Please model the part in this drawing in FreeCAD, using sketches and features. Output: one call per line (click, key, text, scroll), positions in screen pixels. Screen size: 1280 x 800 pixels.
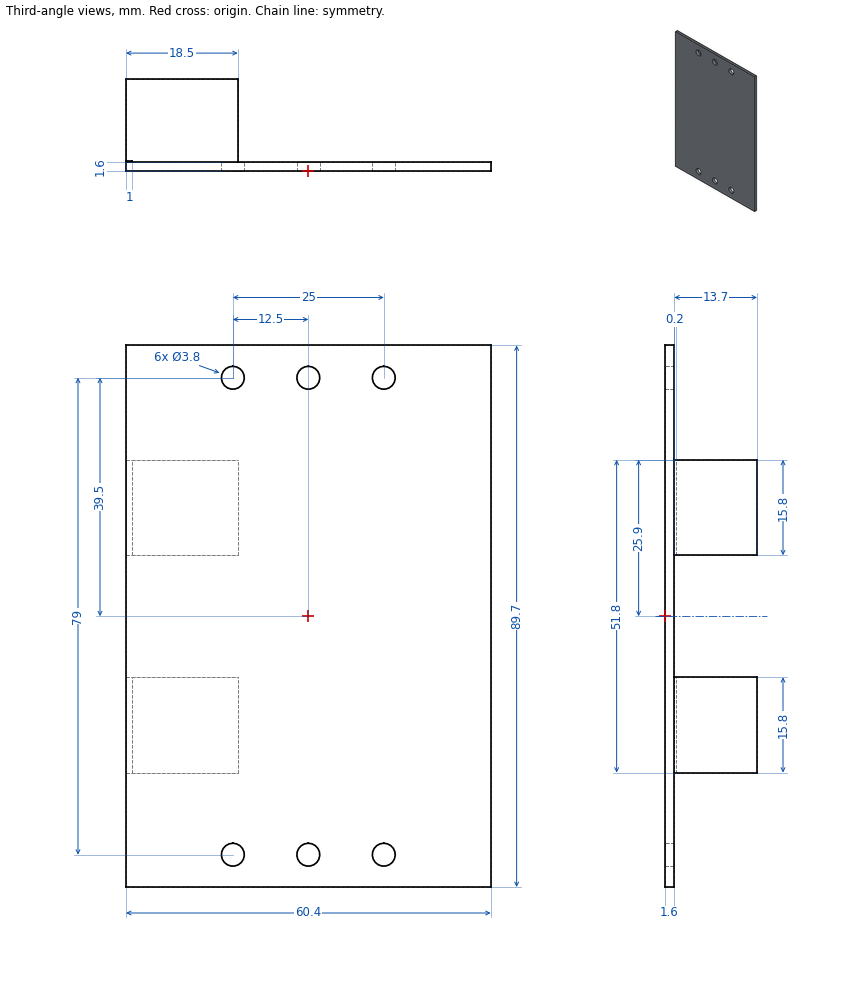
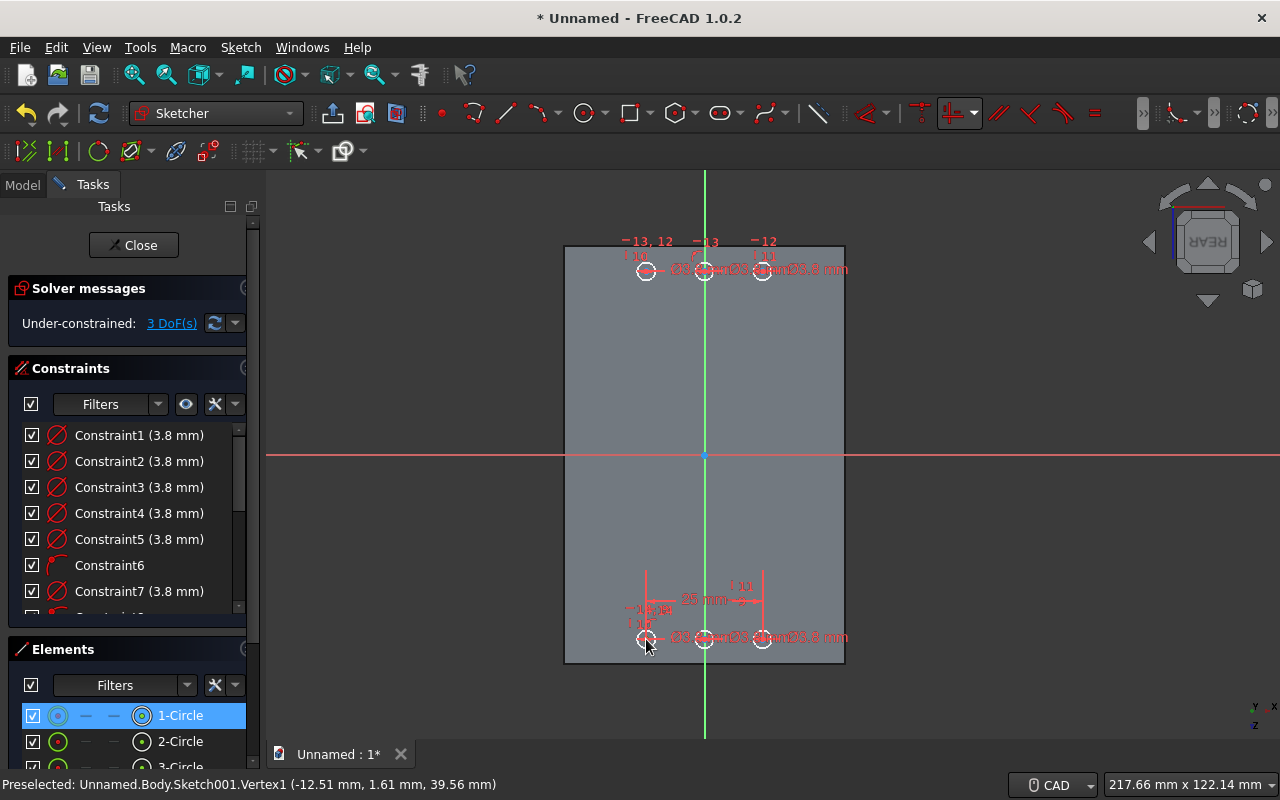
click(646, 271)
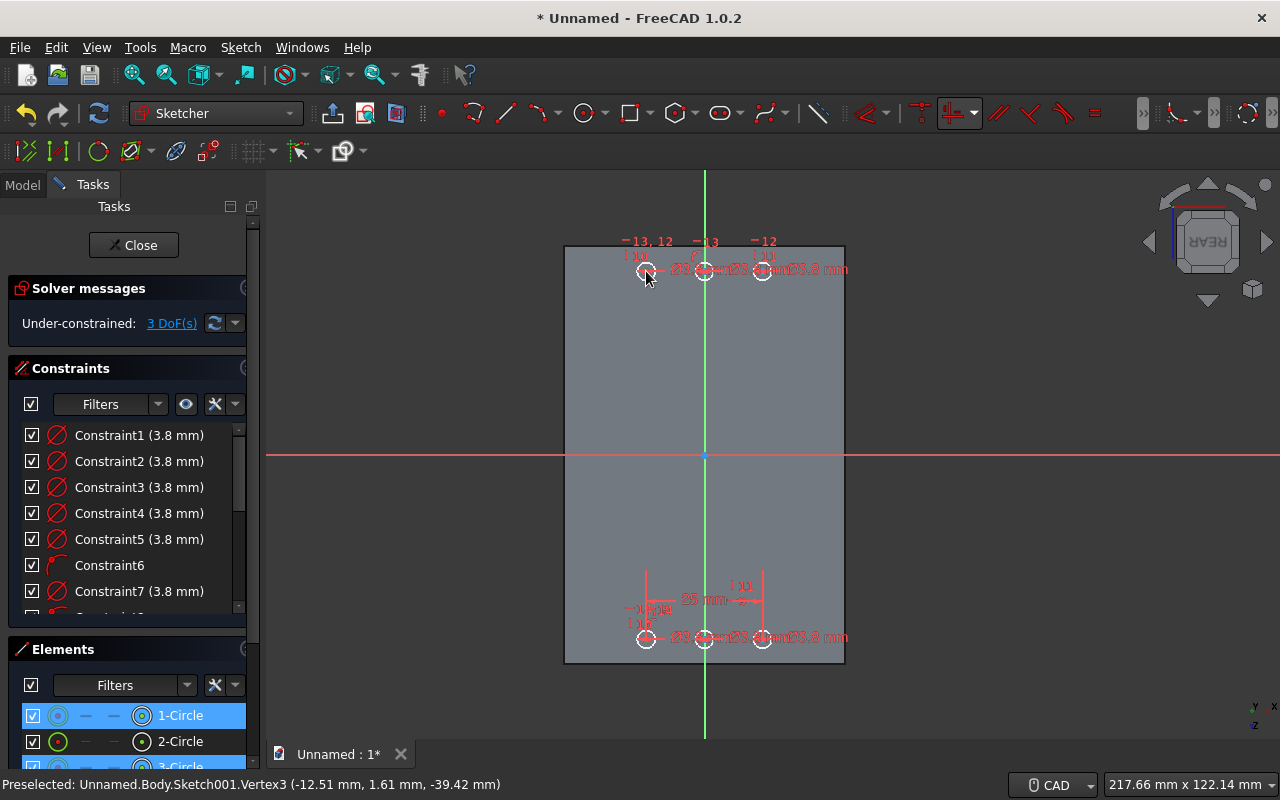
click(888, 114)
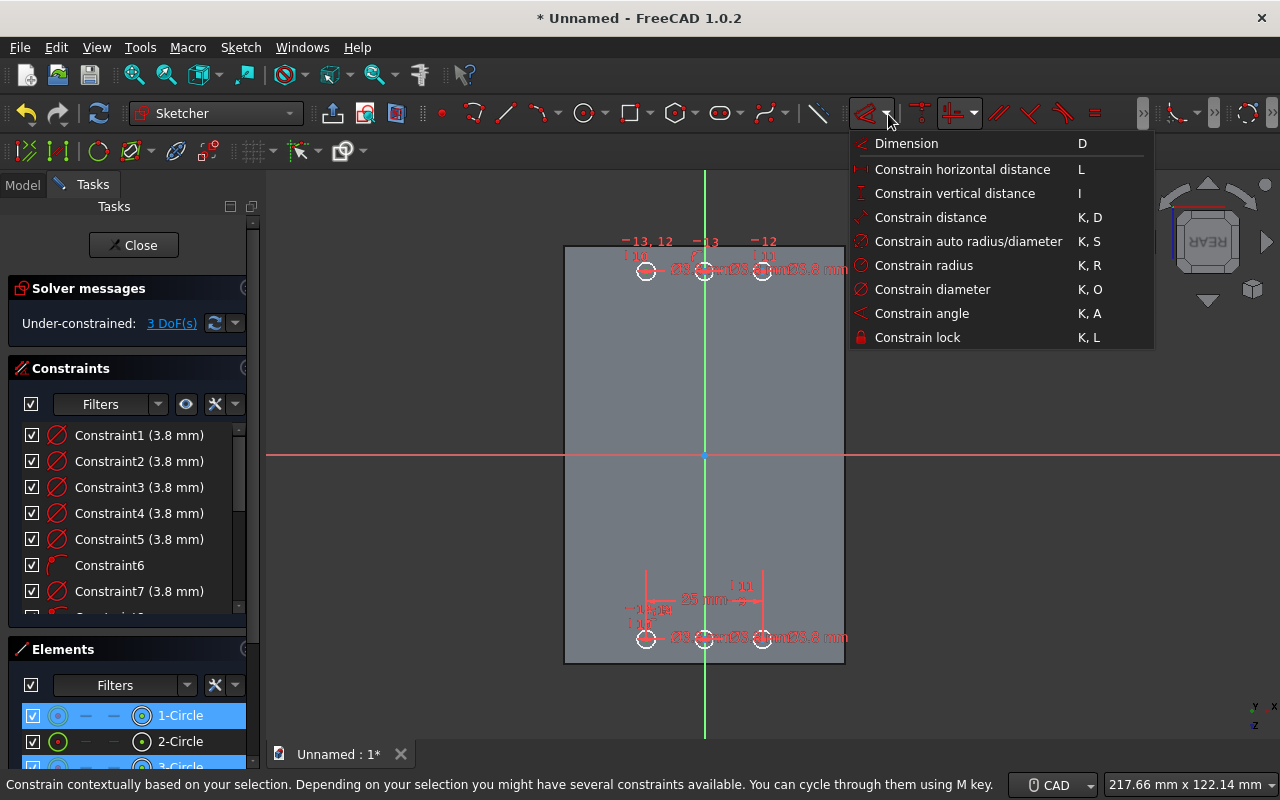
click(1002, 193)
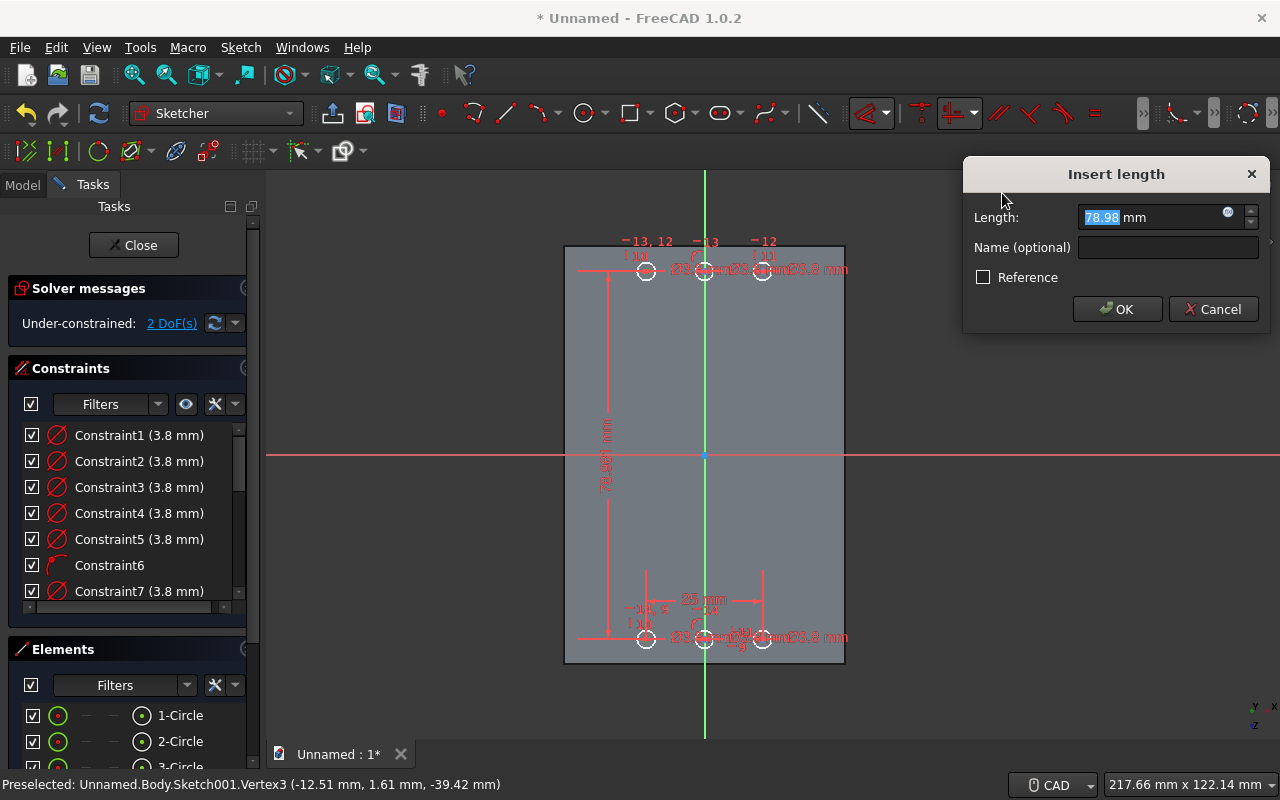
text(79)
key(Return)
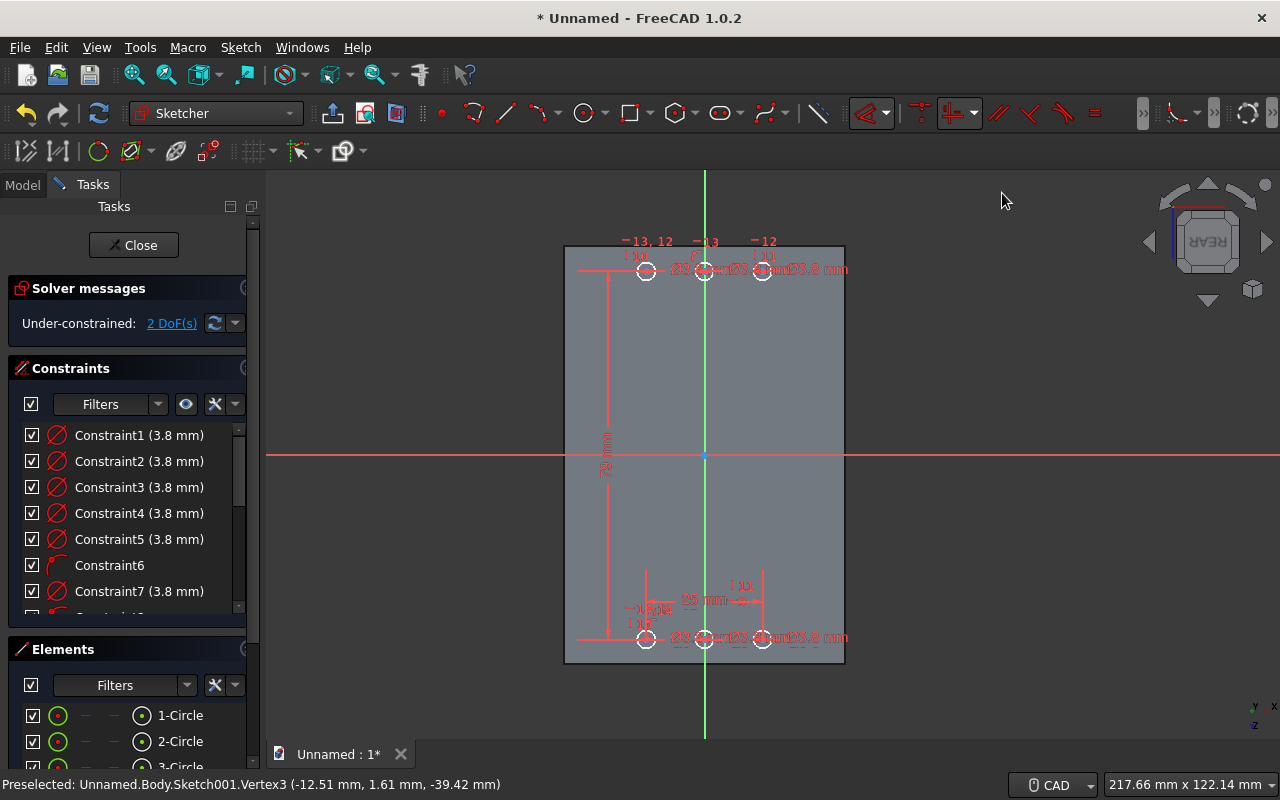
click(646, 640)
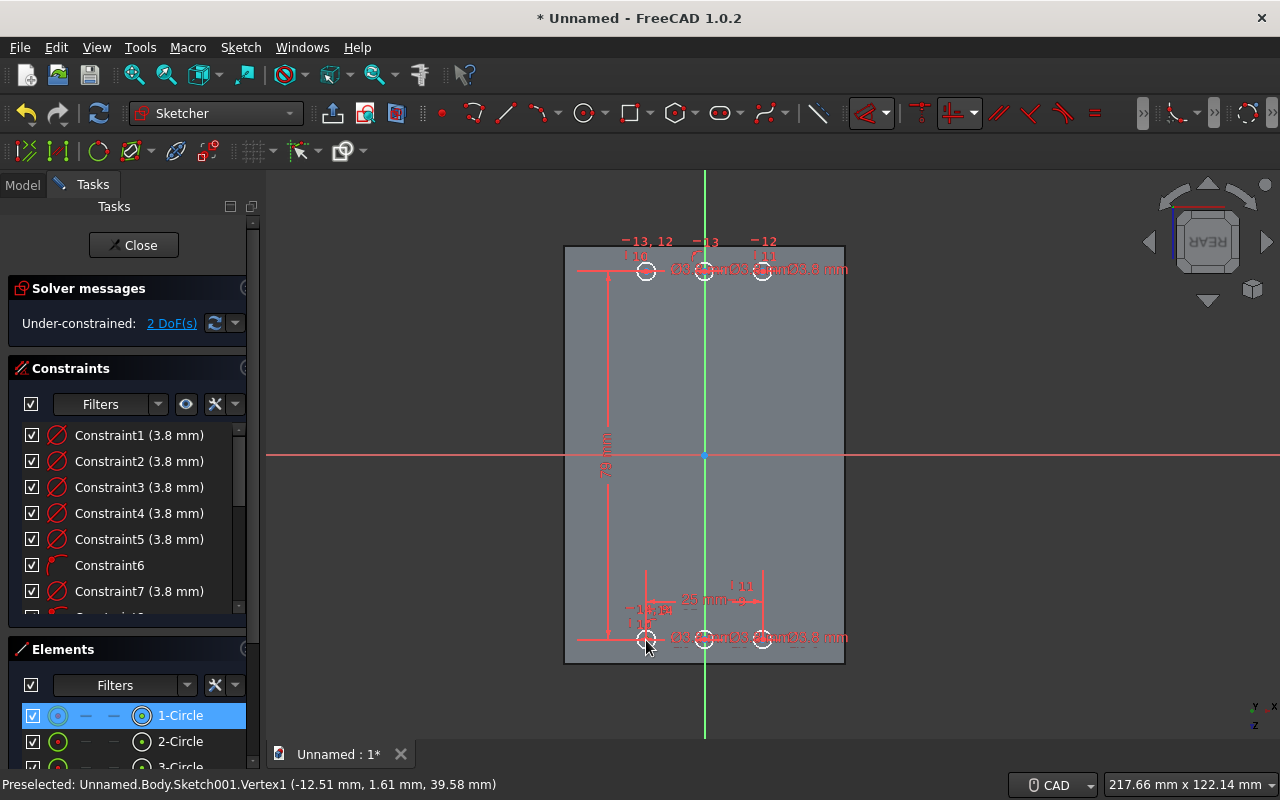
key(l)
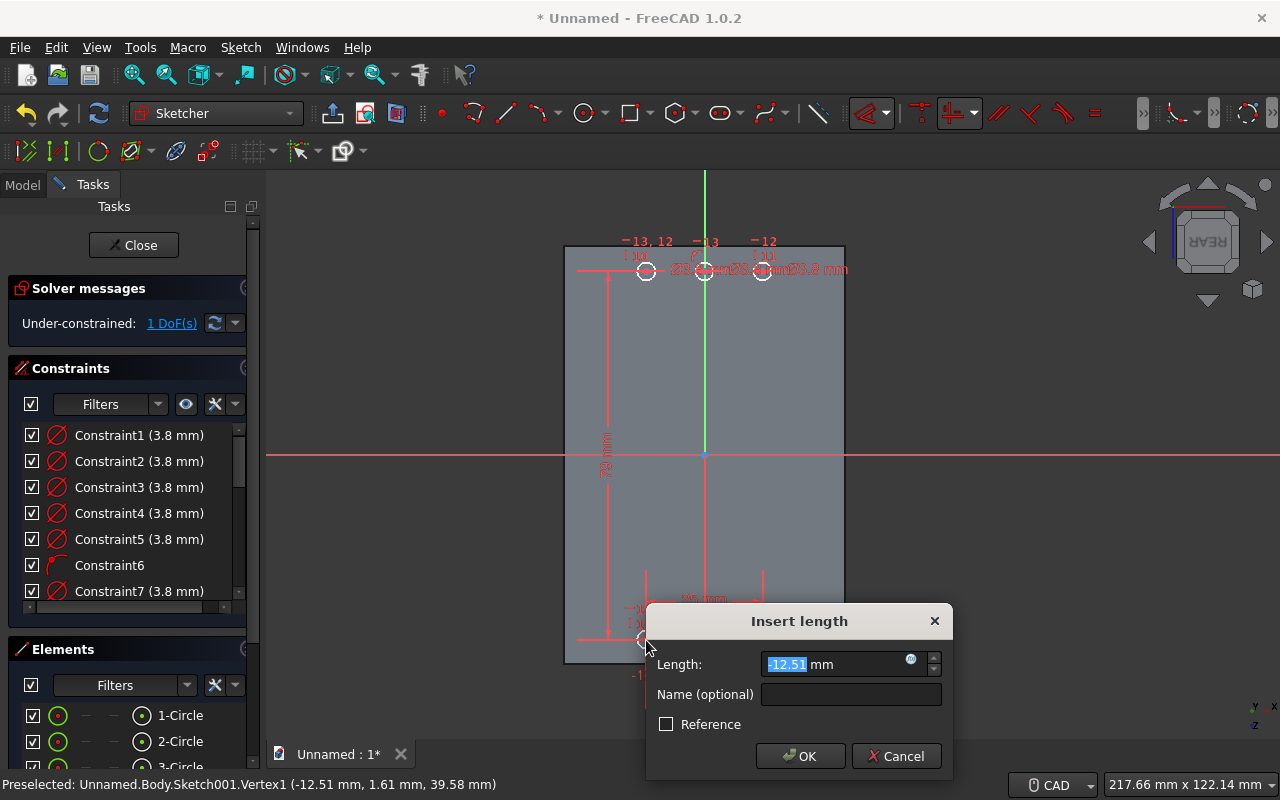
text(-12.5)
key(Return)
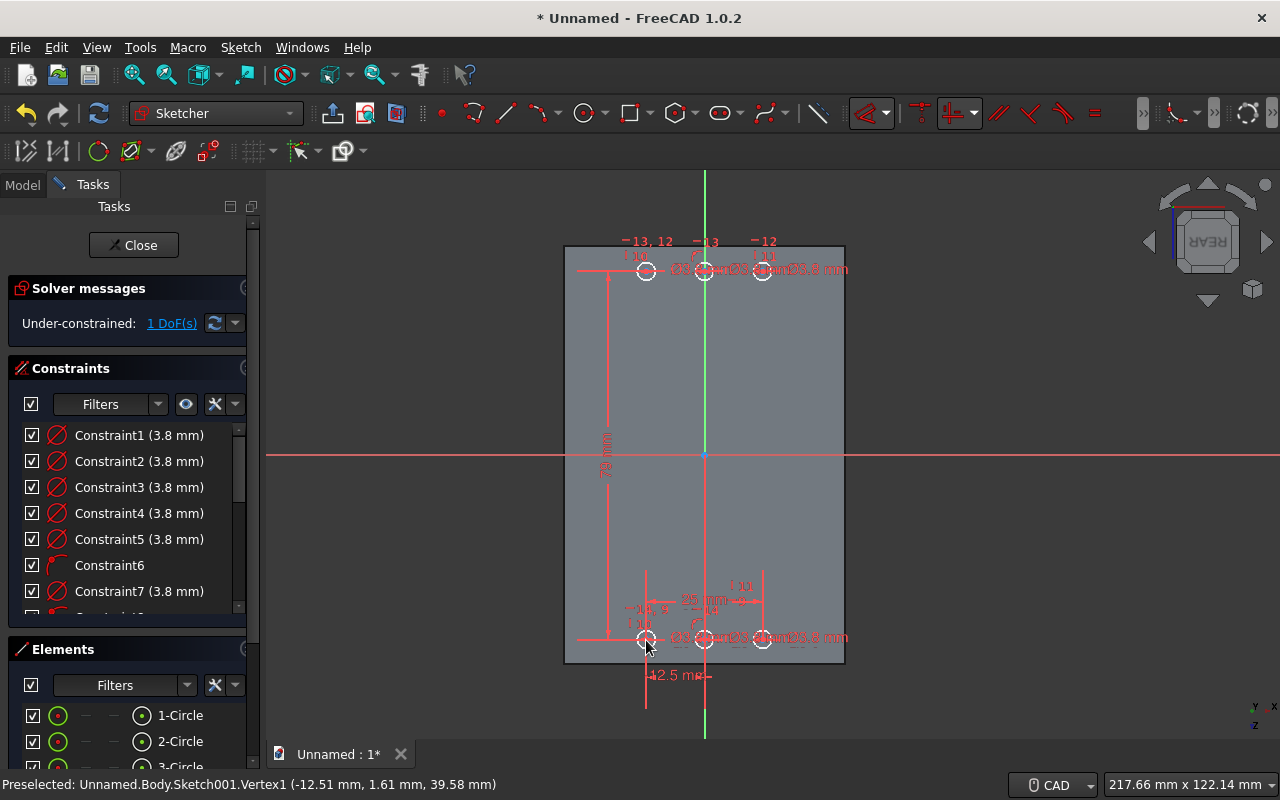
click(646, 640)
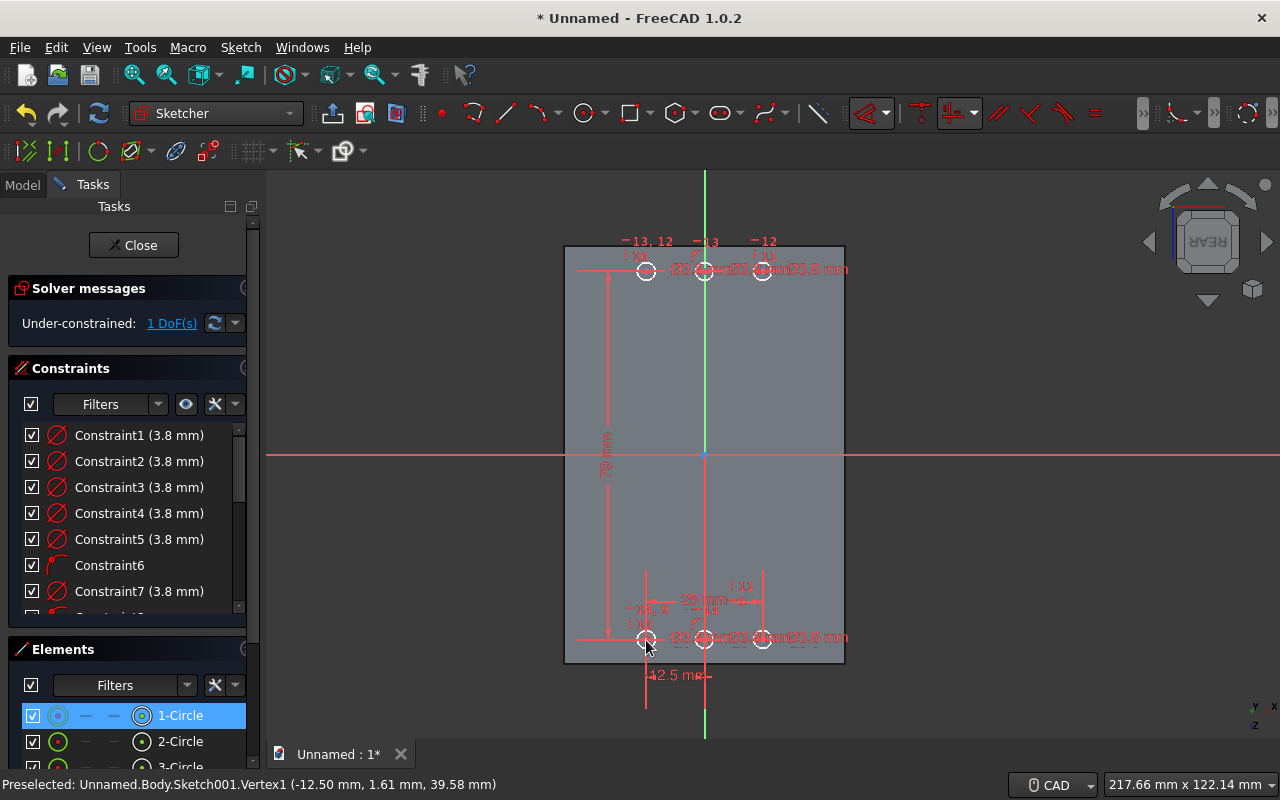
key(i)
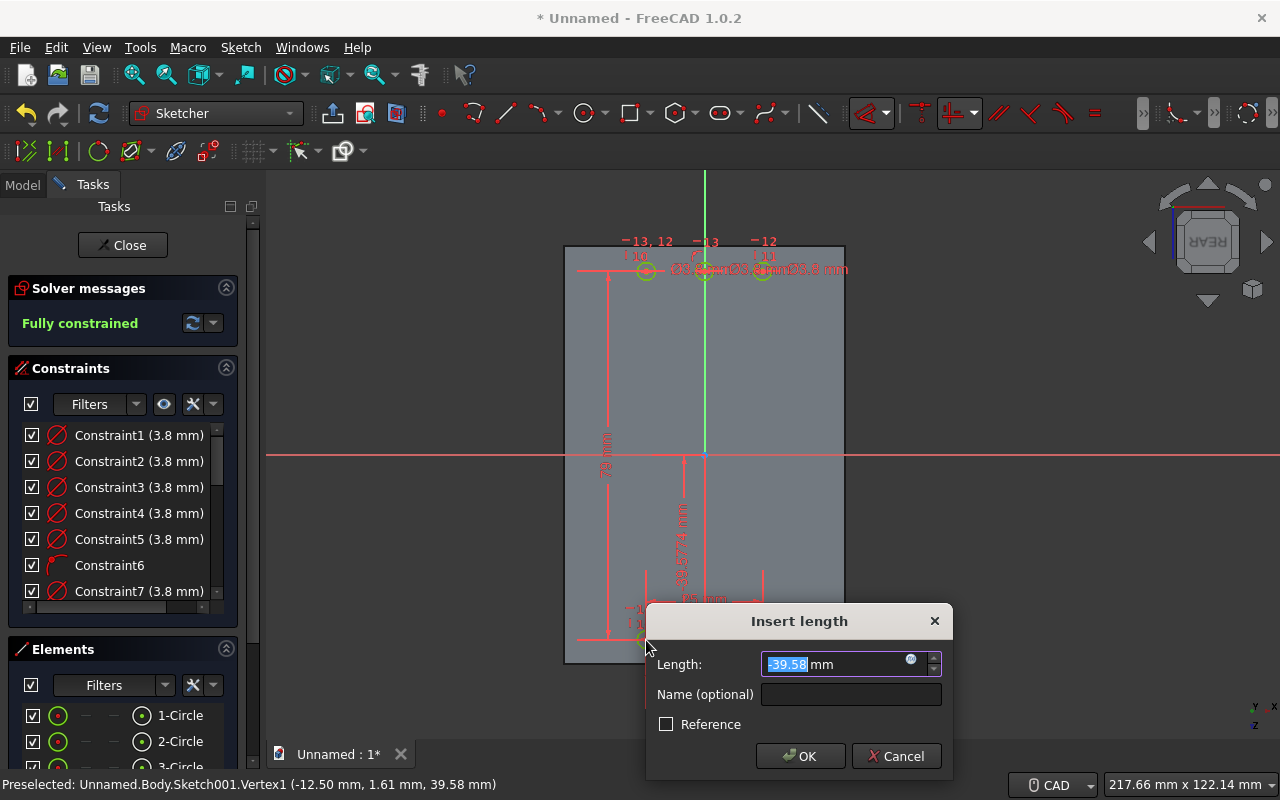
text(-39.5)
key(Return)